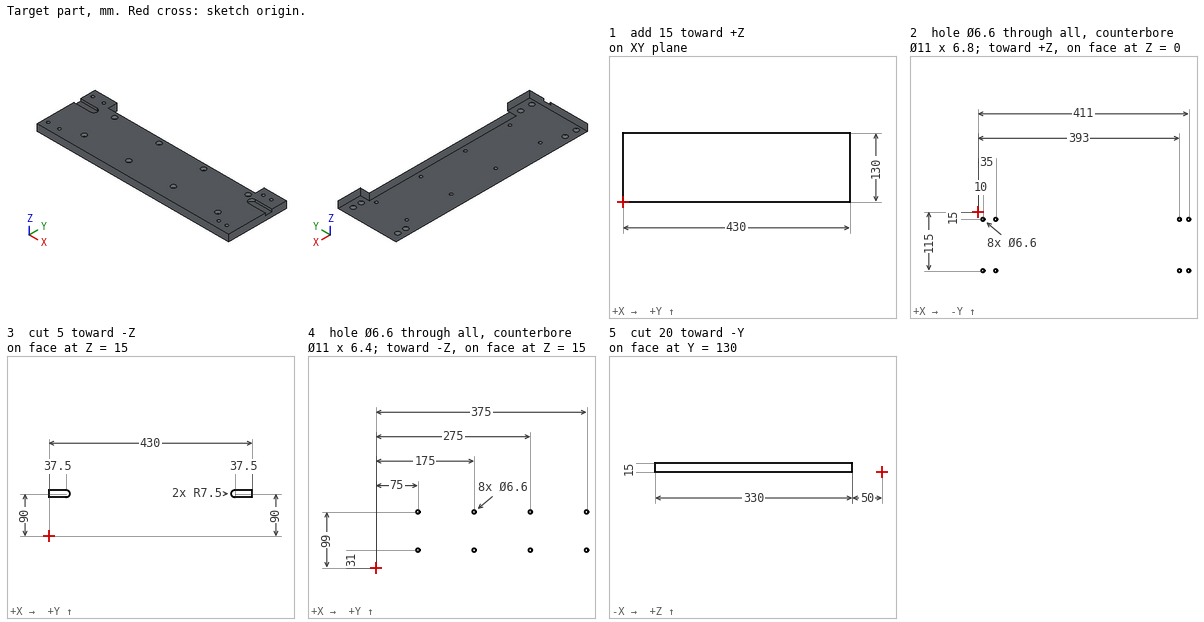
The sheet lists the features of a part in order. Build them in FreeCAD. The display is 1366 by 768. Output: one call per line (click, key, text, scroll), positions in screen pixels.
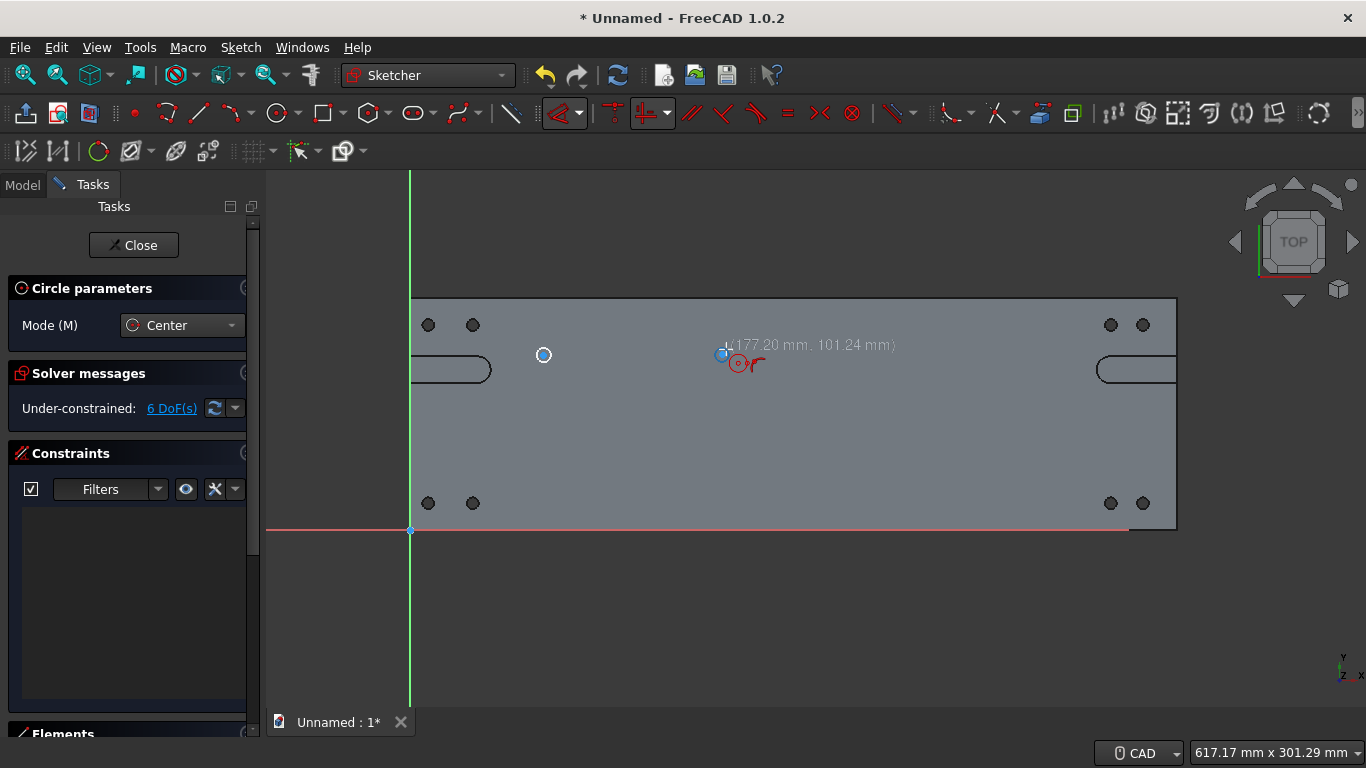
scroll(544, 475, up, 7)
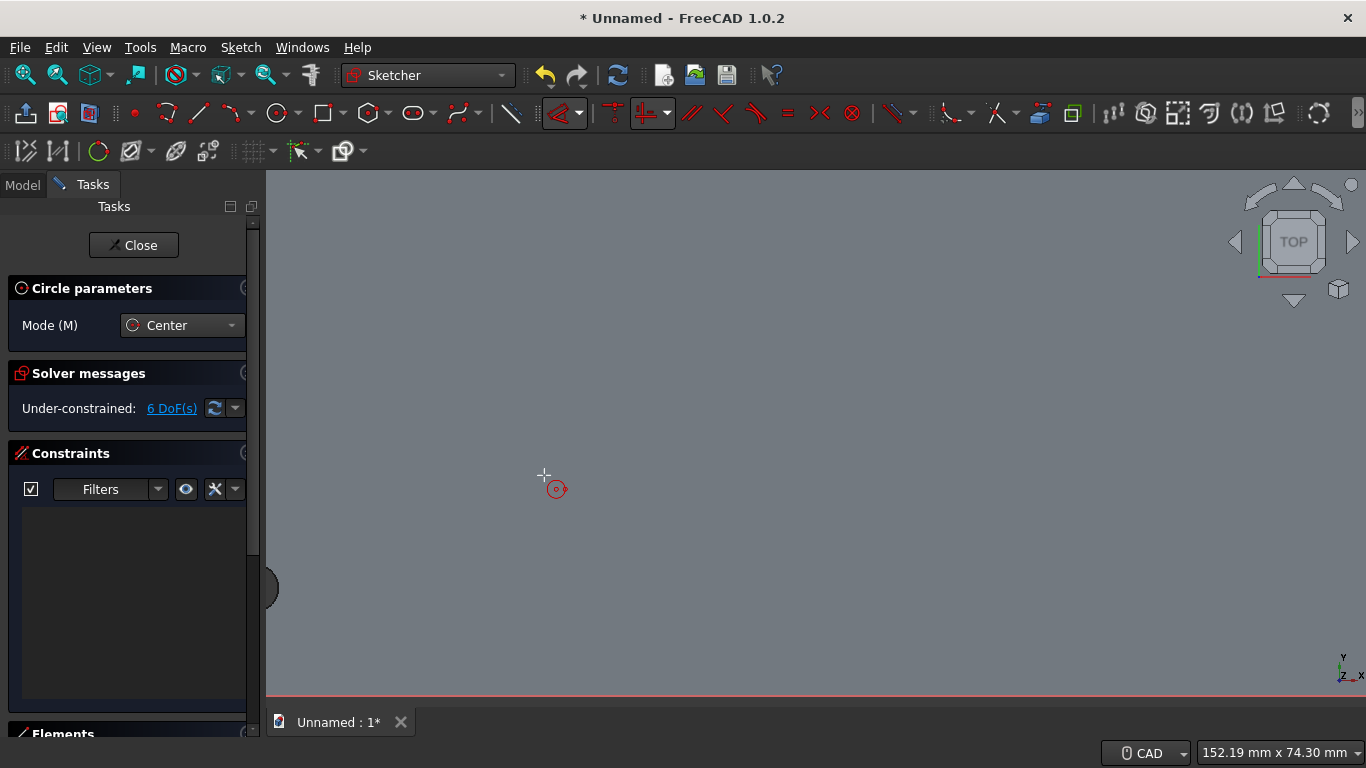
scroll(544, 475, down, 7)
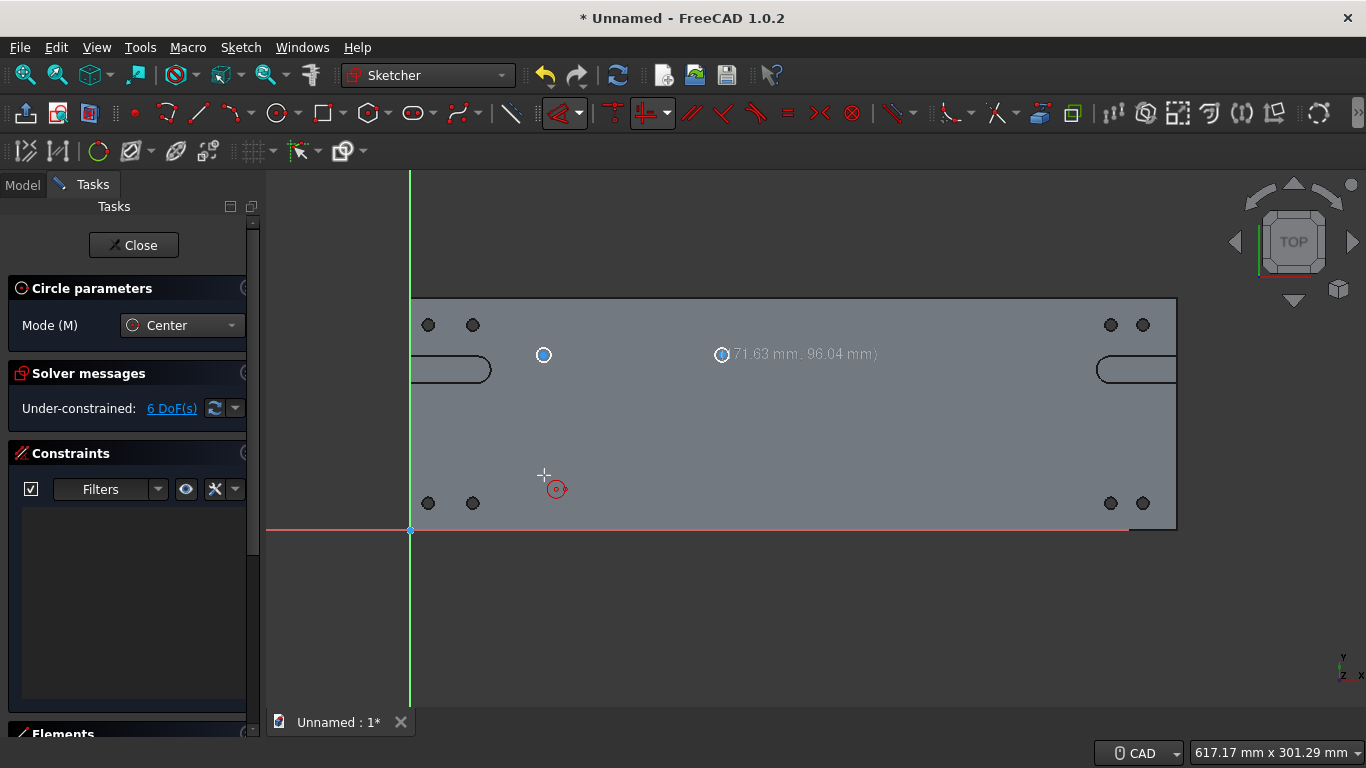
click(544, 475)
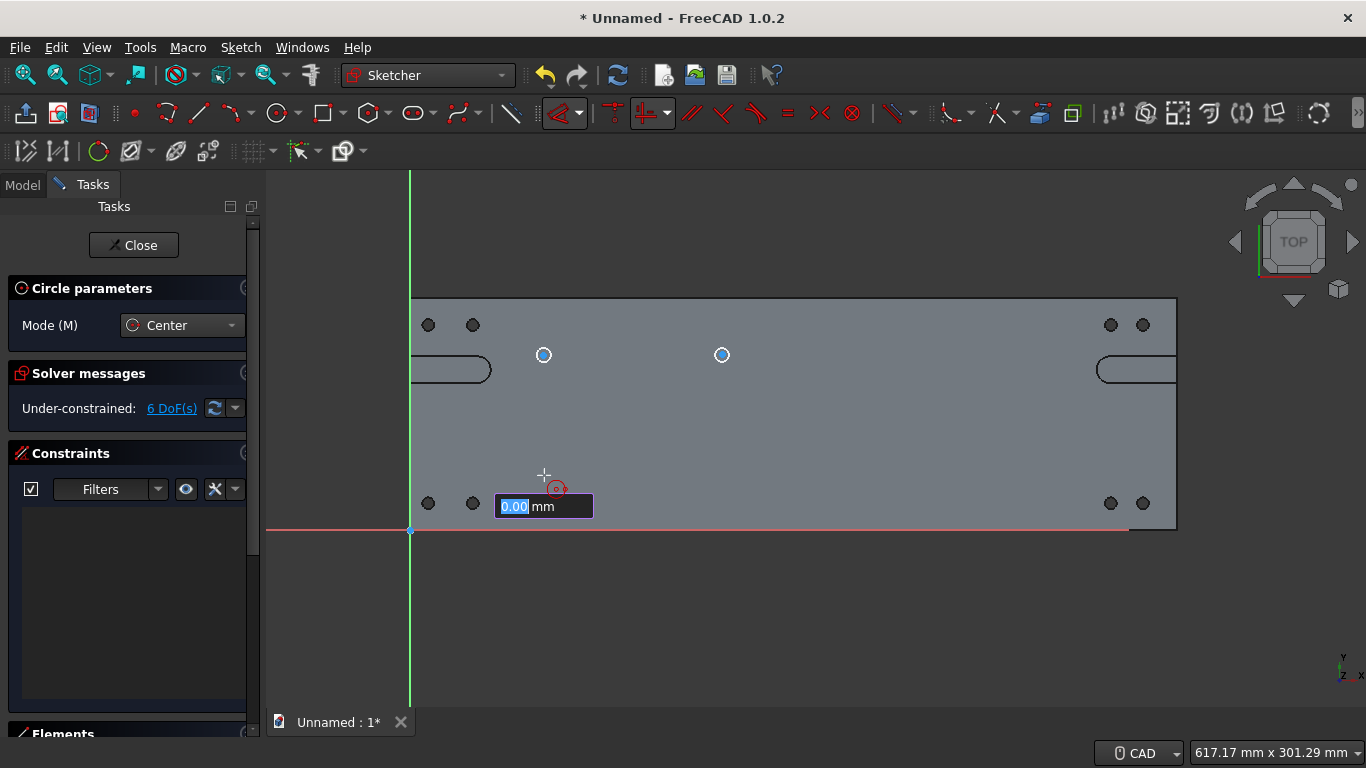
scroll(548, 471, up, 5)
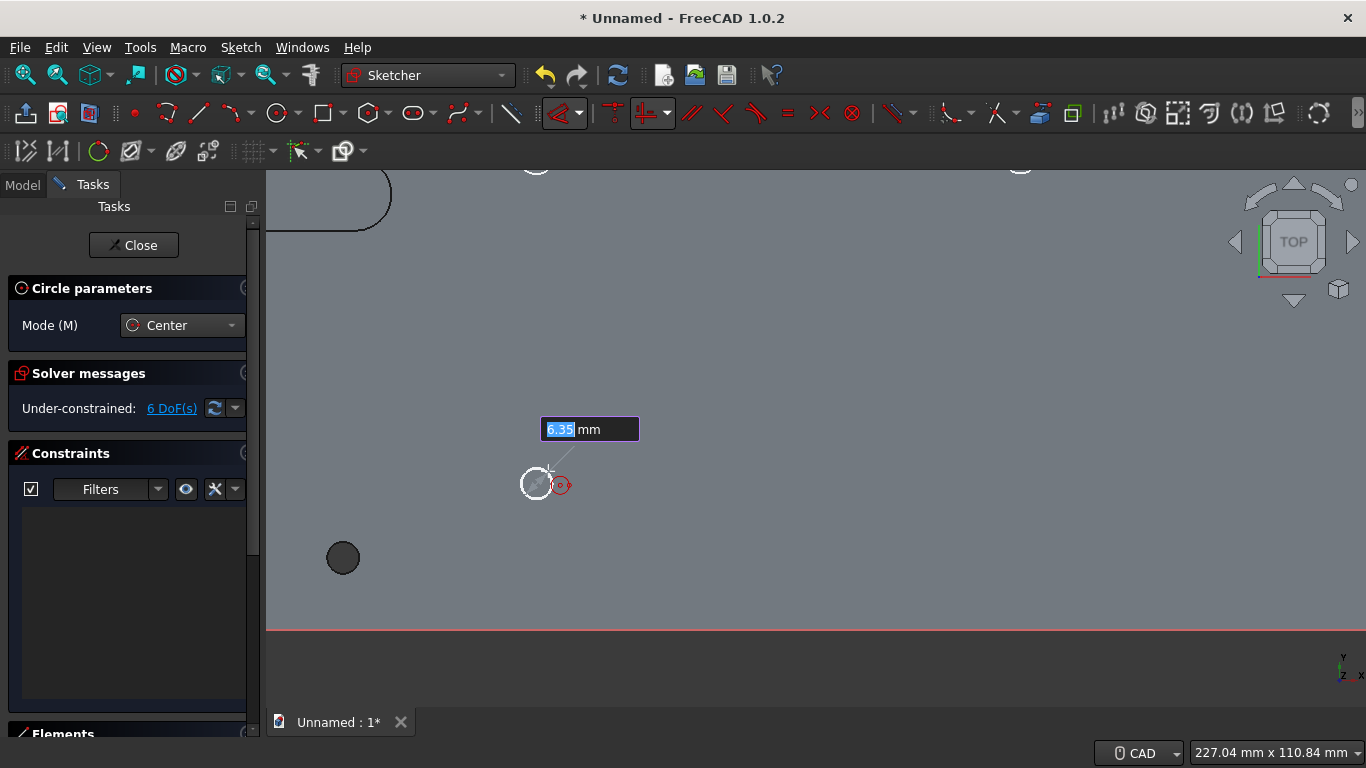
click(548, 469)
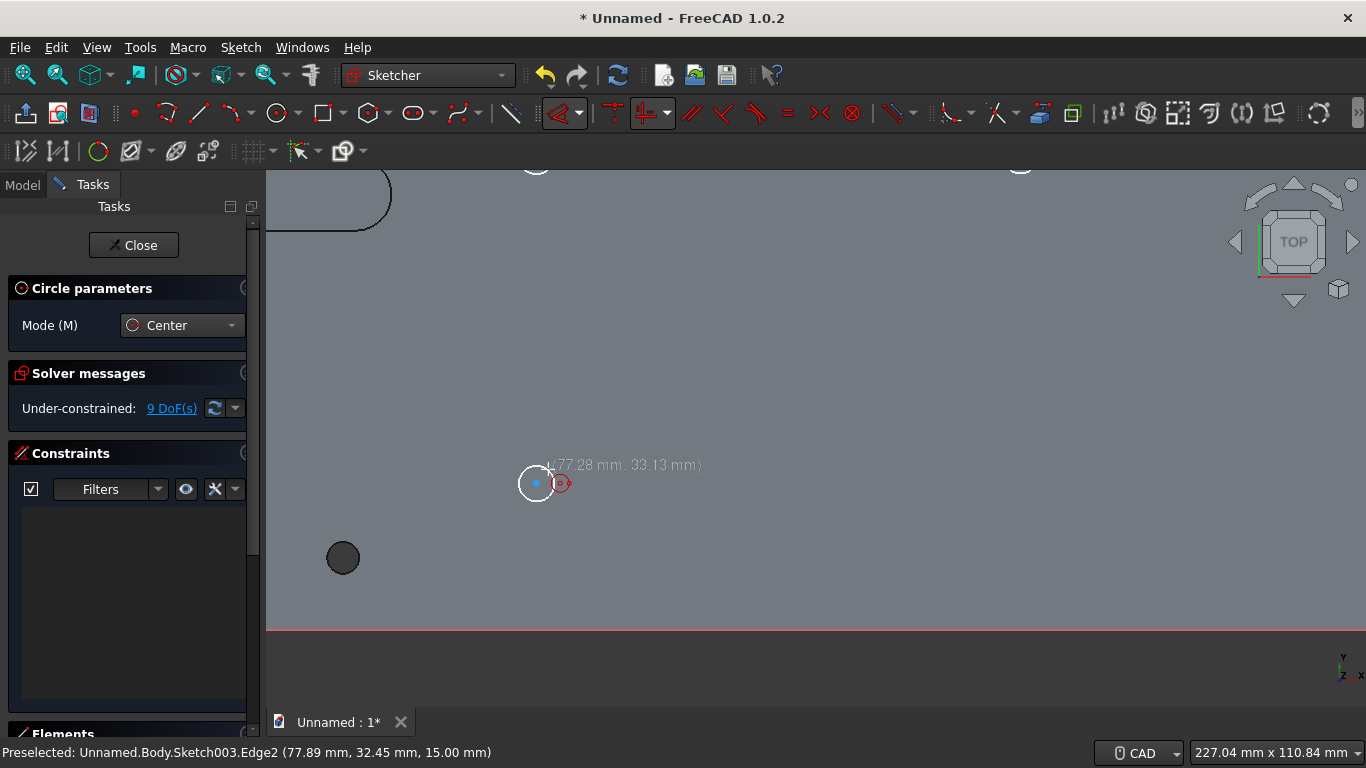
scroll(1021, 480, up, 2)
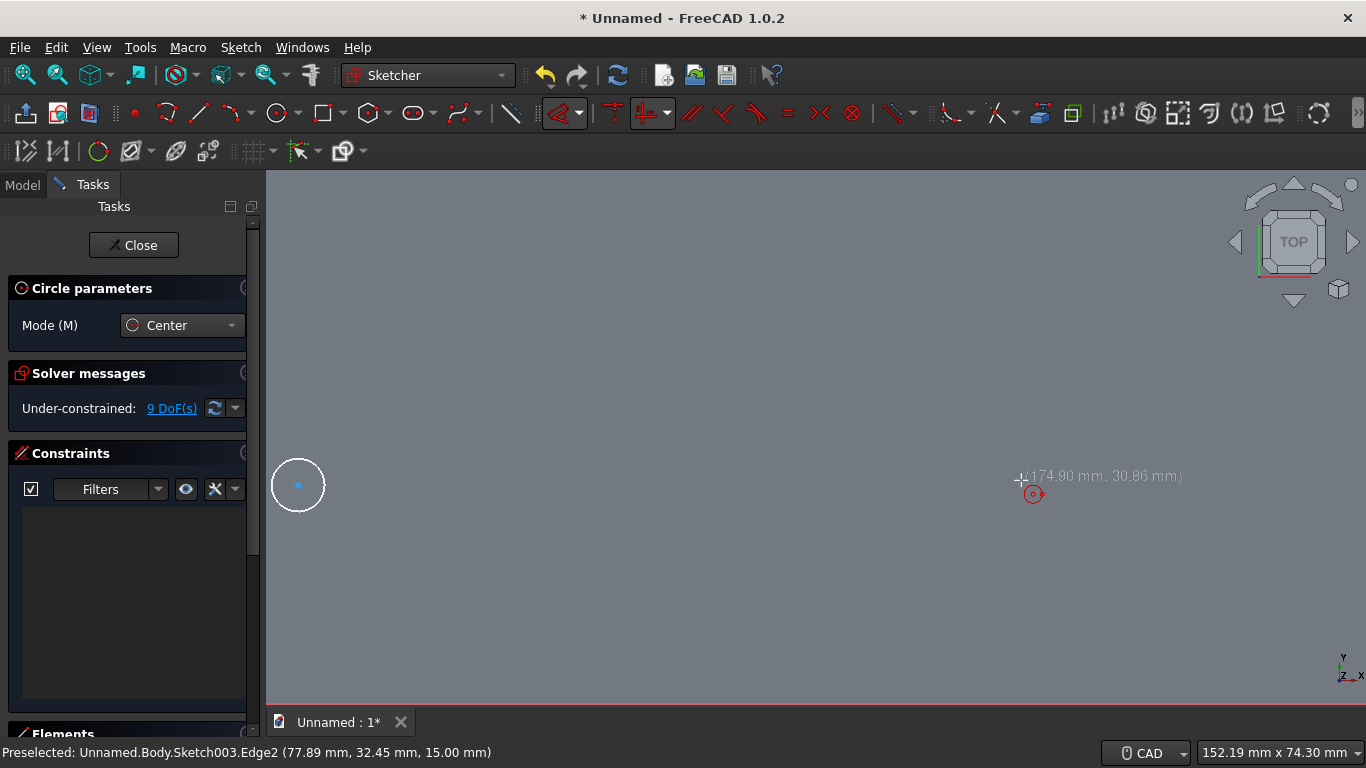
scroll(624, 473, down, 7)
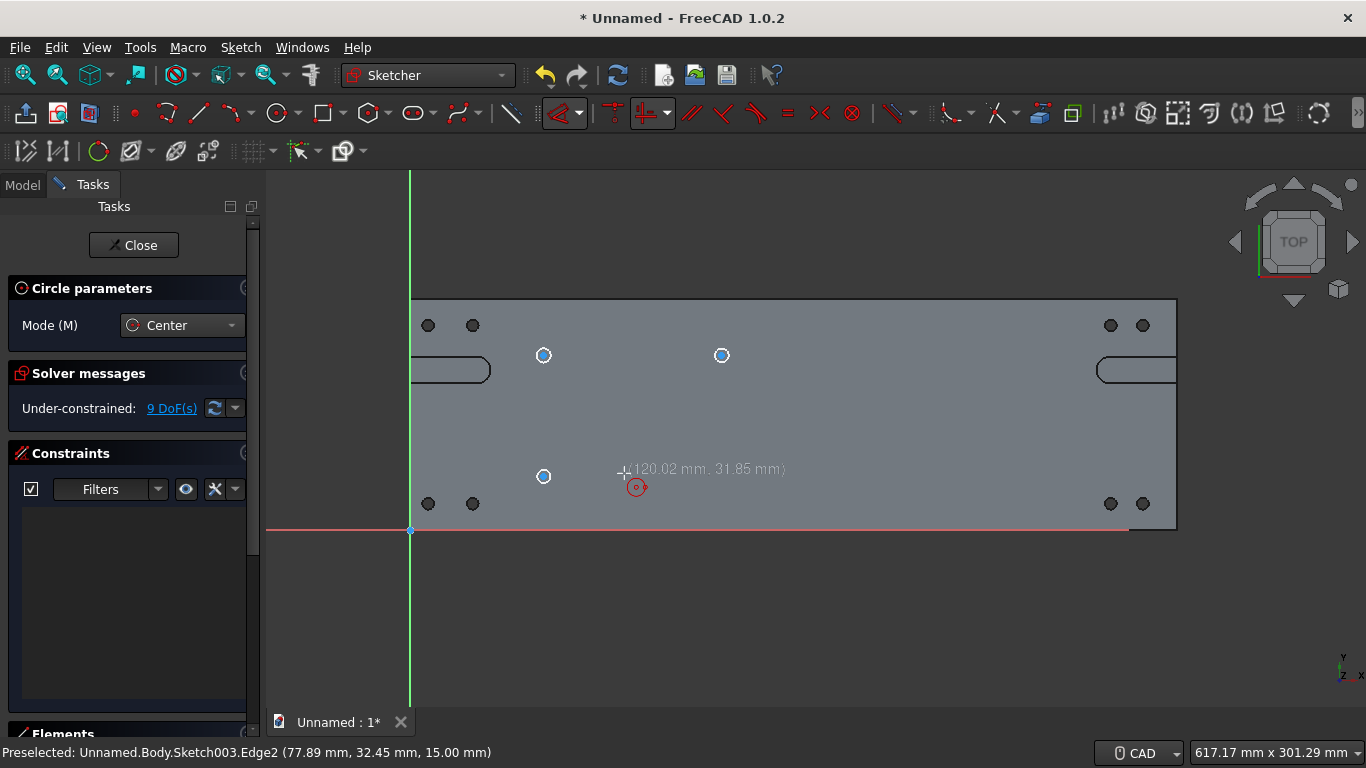
click(722, 475)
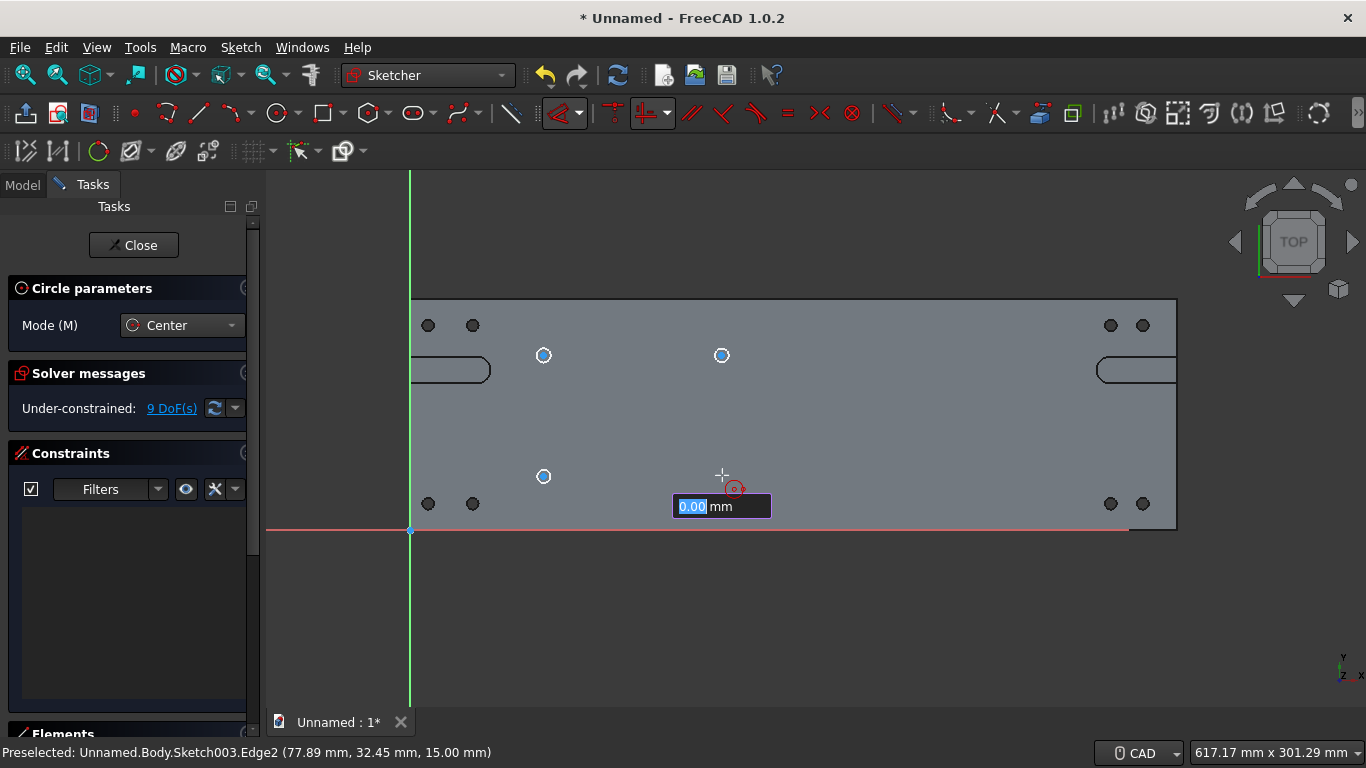
scroll(726, 471, up, 5)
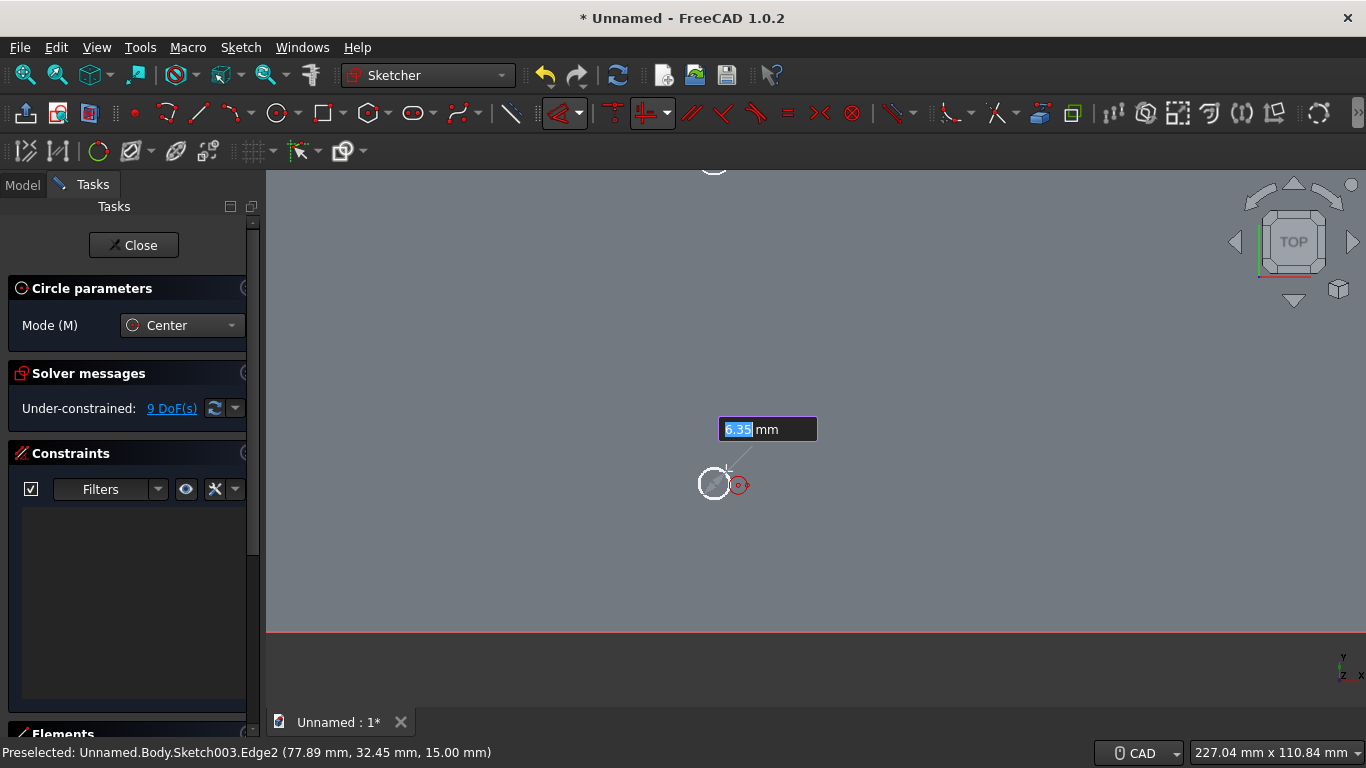
click(726, 470)